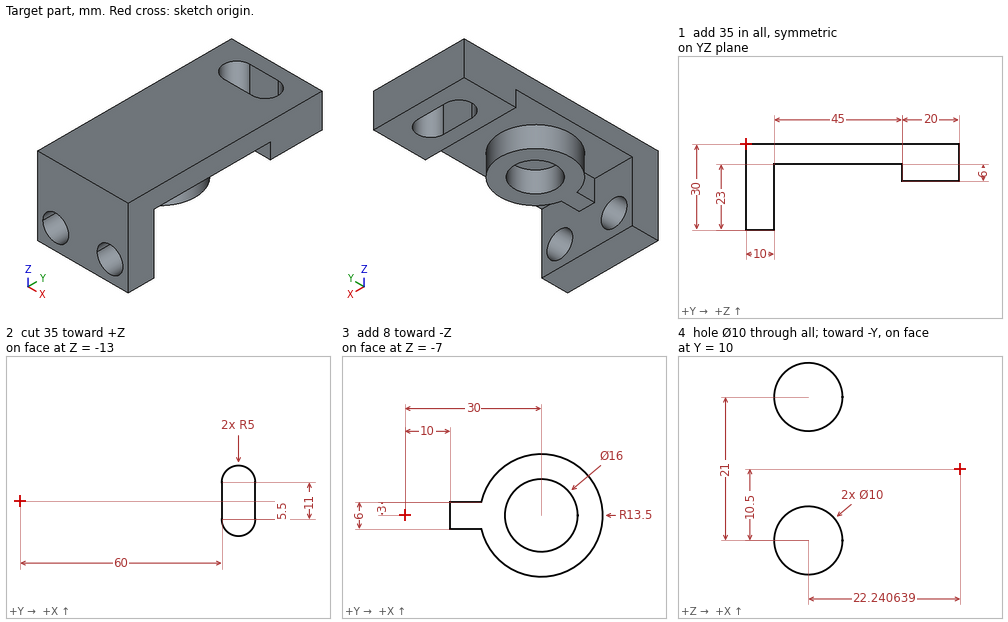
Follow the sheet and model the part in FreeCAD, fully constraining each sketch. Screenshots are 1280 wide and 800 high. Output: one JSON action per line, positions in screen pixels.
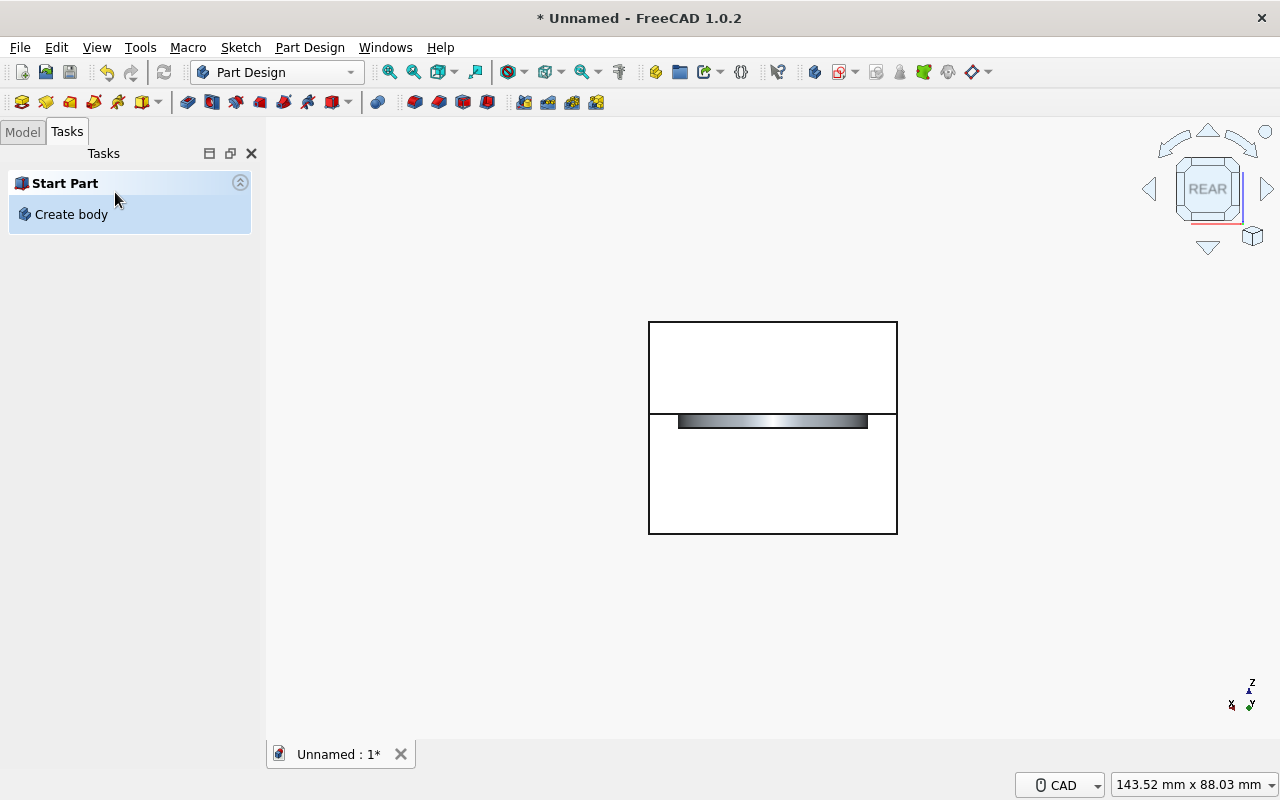
{"action": "key", "text": "v f"}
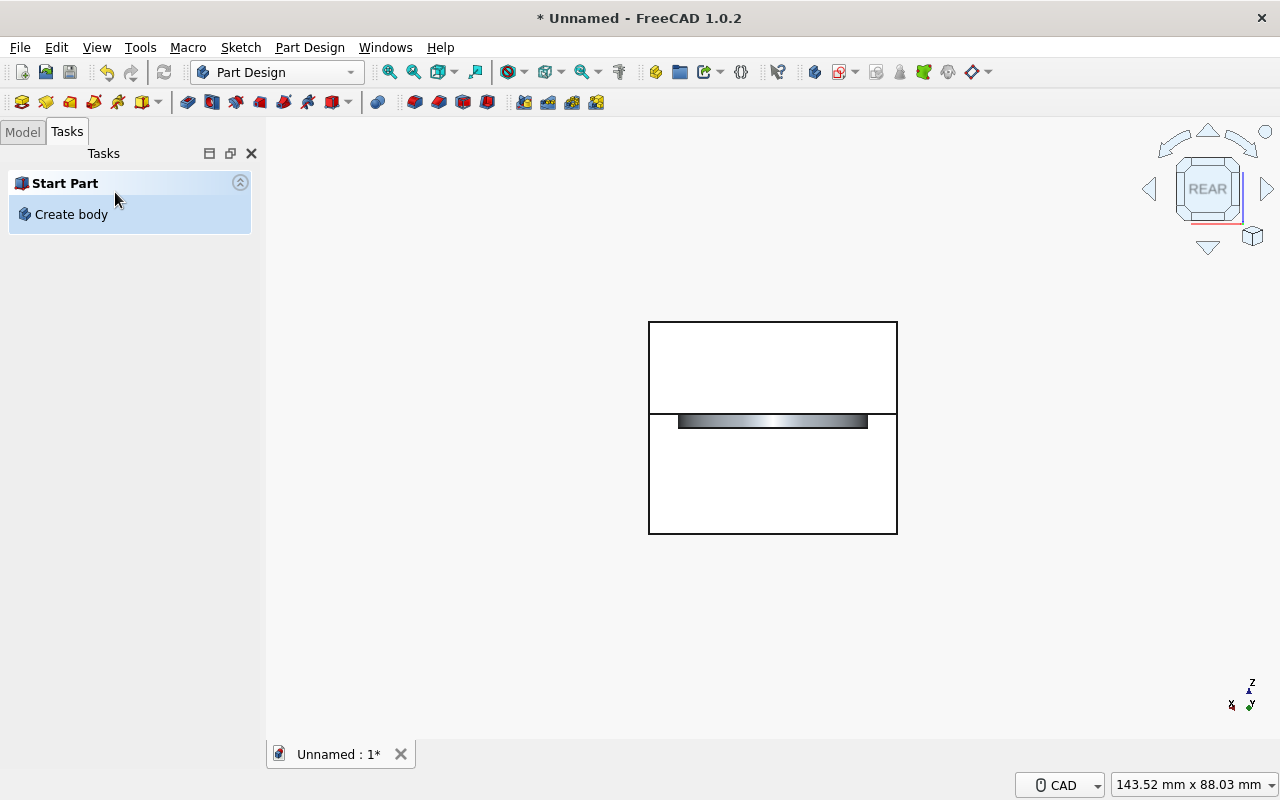
{"action": "left_click", "coordinate": [844, 475]}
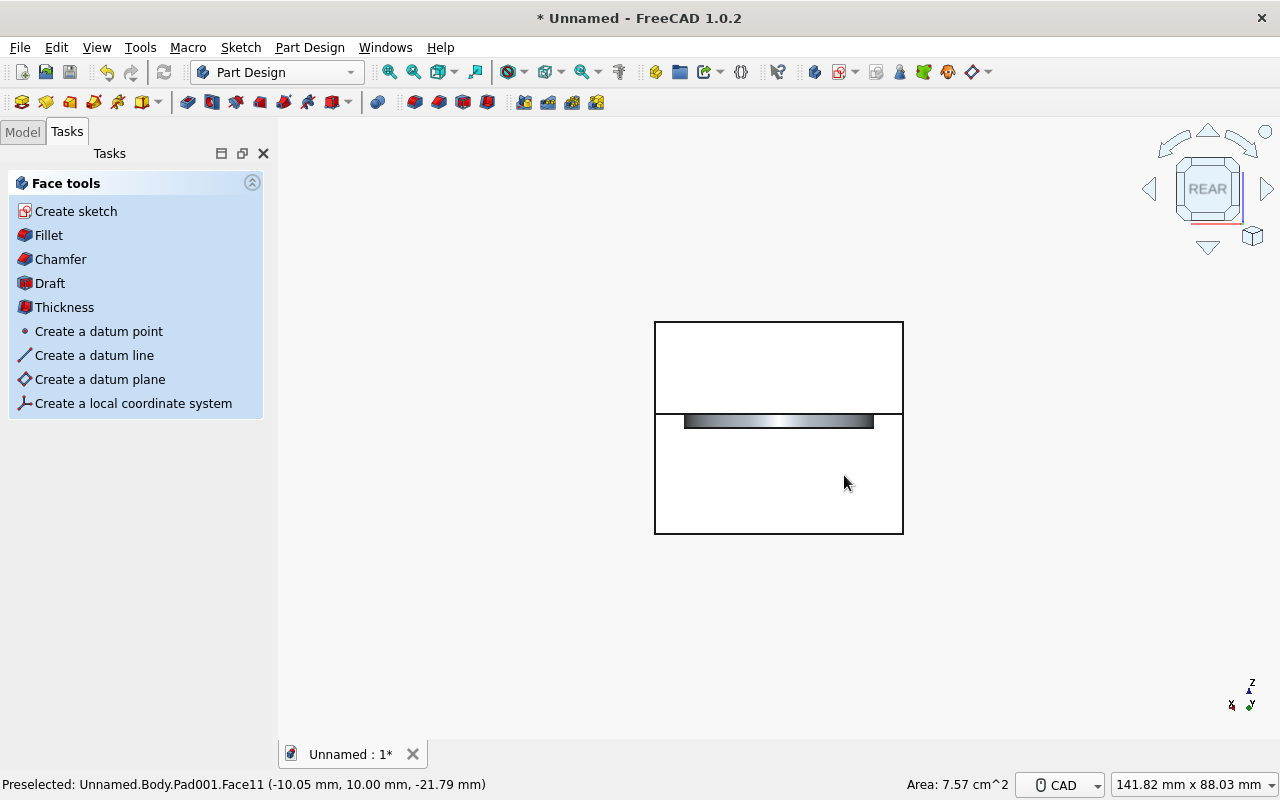
{"action": "left_click", "coordinate": [840, 72]}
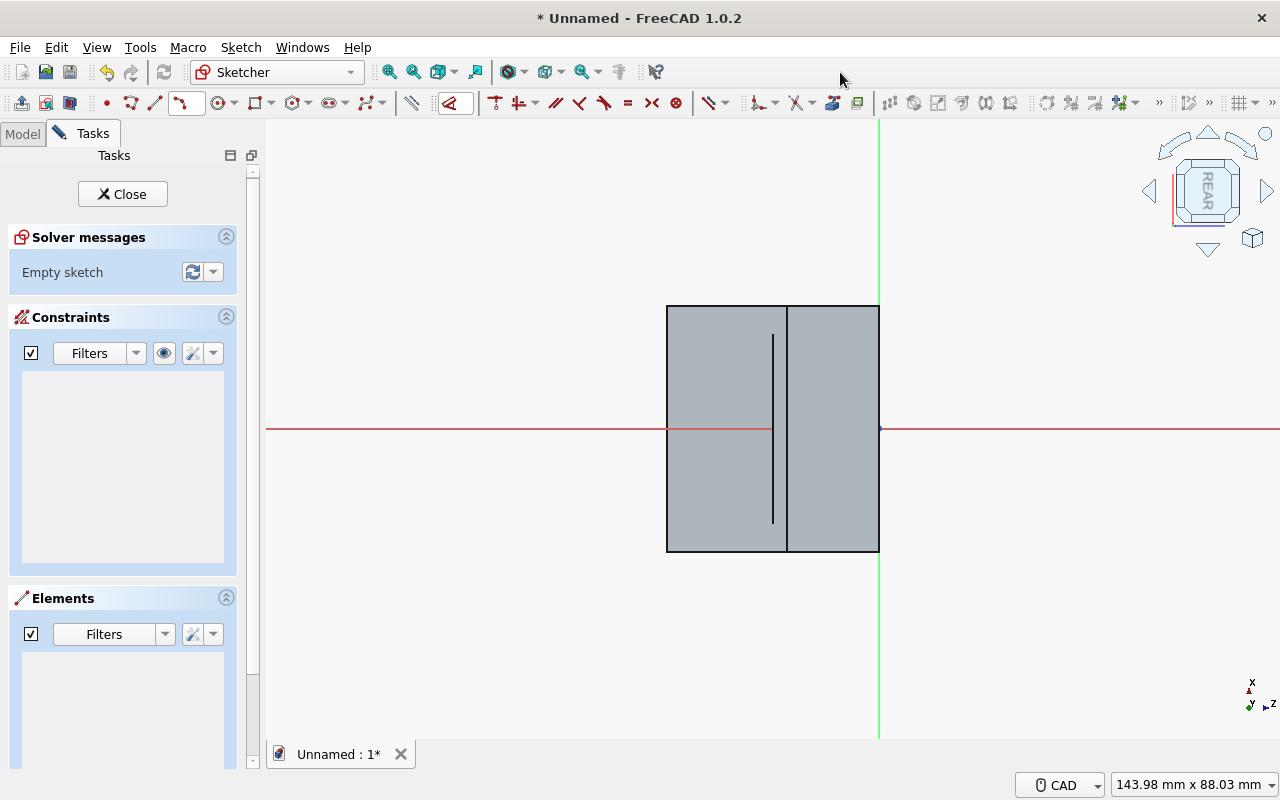
{"action": "left_click", "coordinate": [70, 104]}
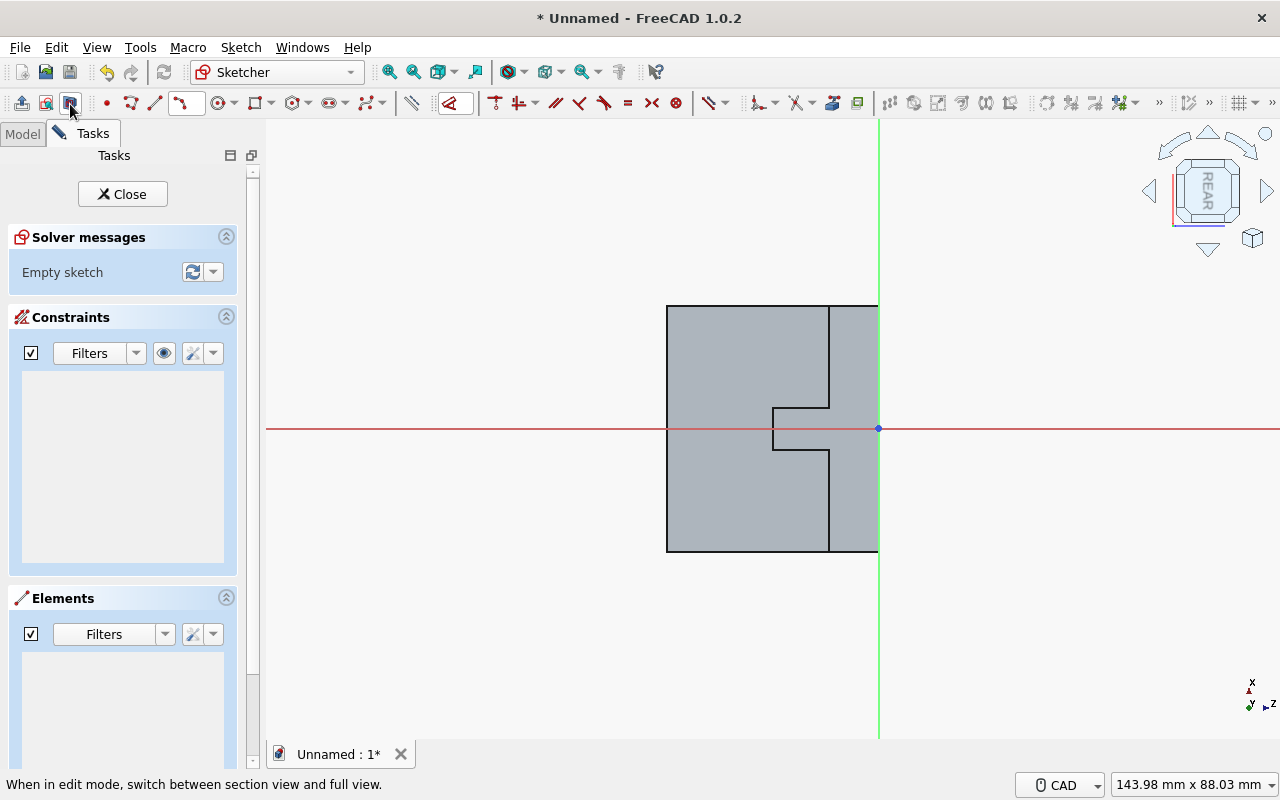
{"action": "scroll", "coordinate": [878, 429], "scroll_direction": "up", "scroll_amount": 3}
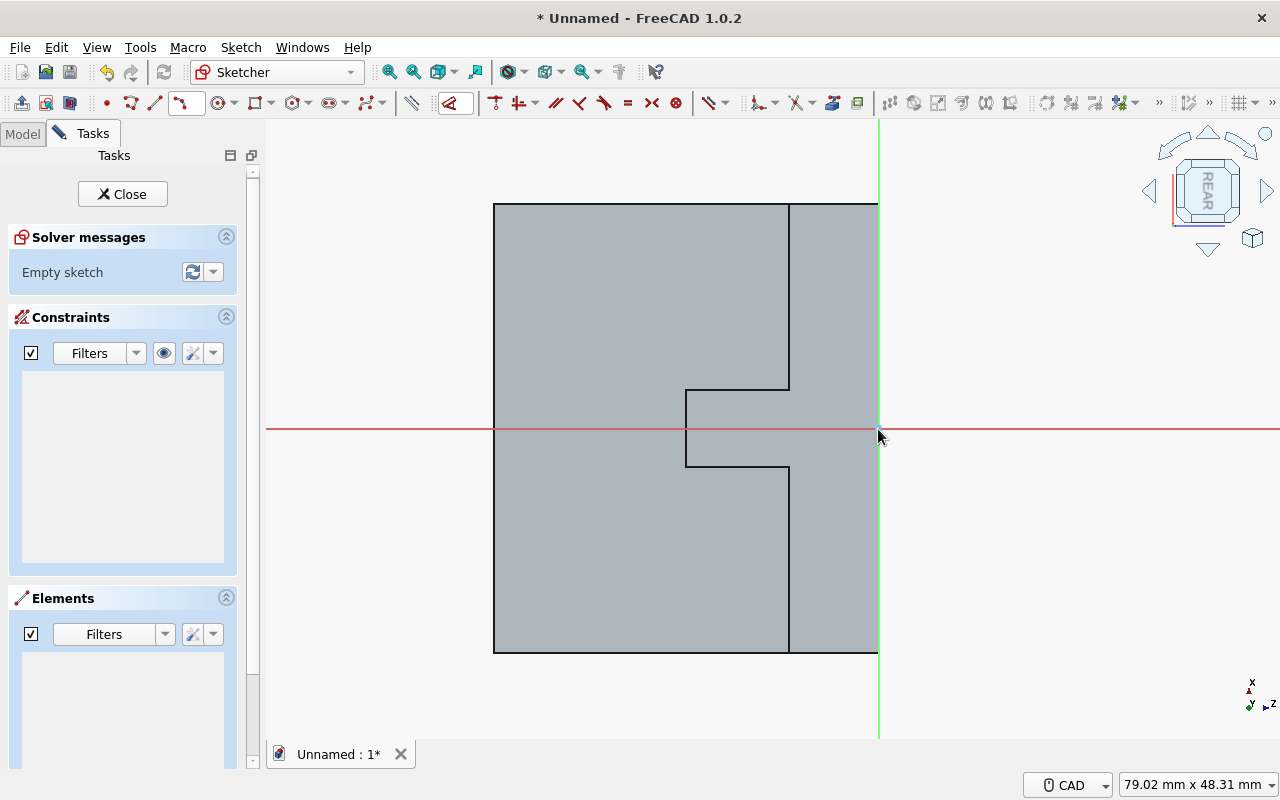
{"action": "left_click", "coordinate": [218, 104]}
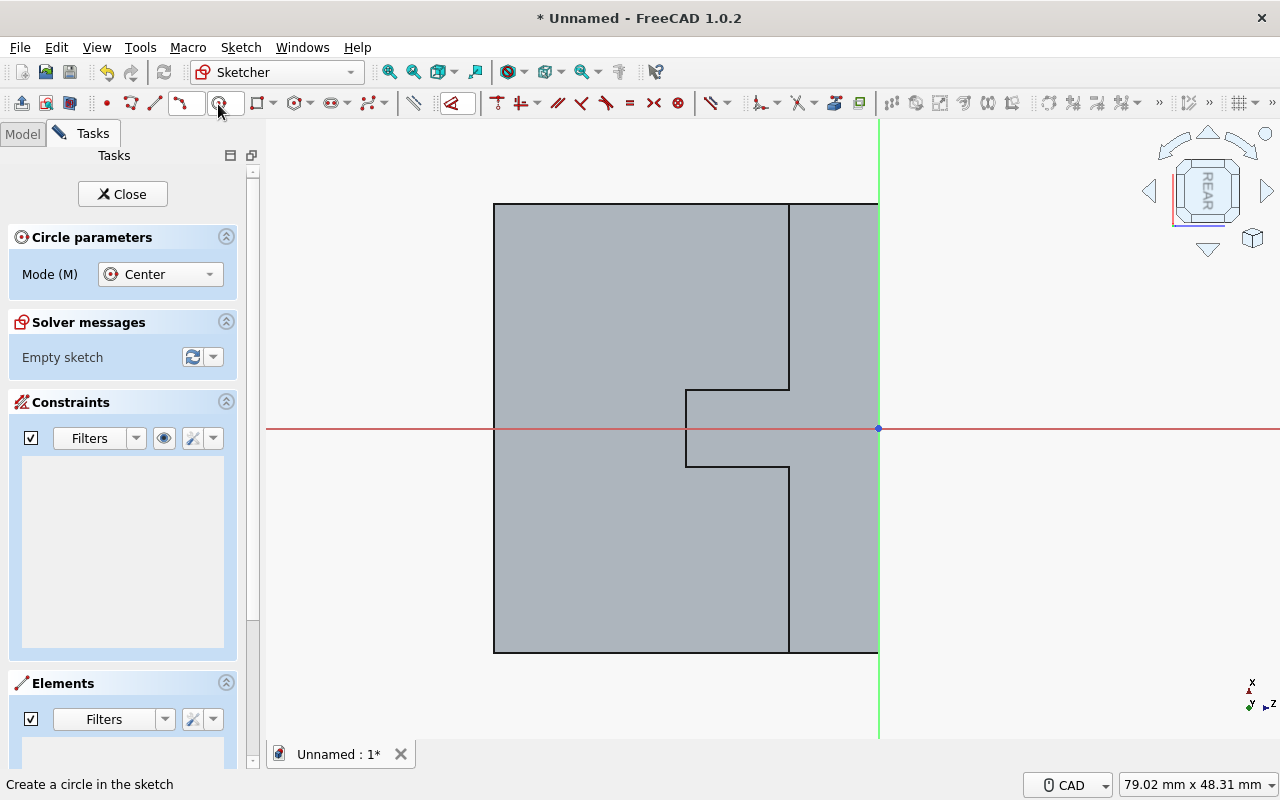
{"action": "left_click", "coordinate": [593, 563]}
{"action": "mouse_move", "coordinate": [639, 518]}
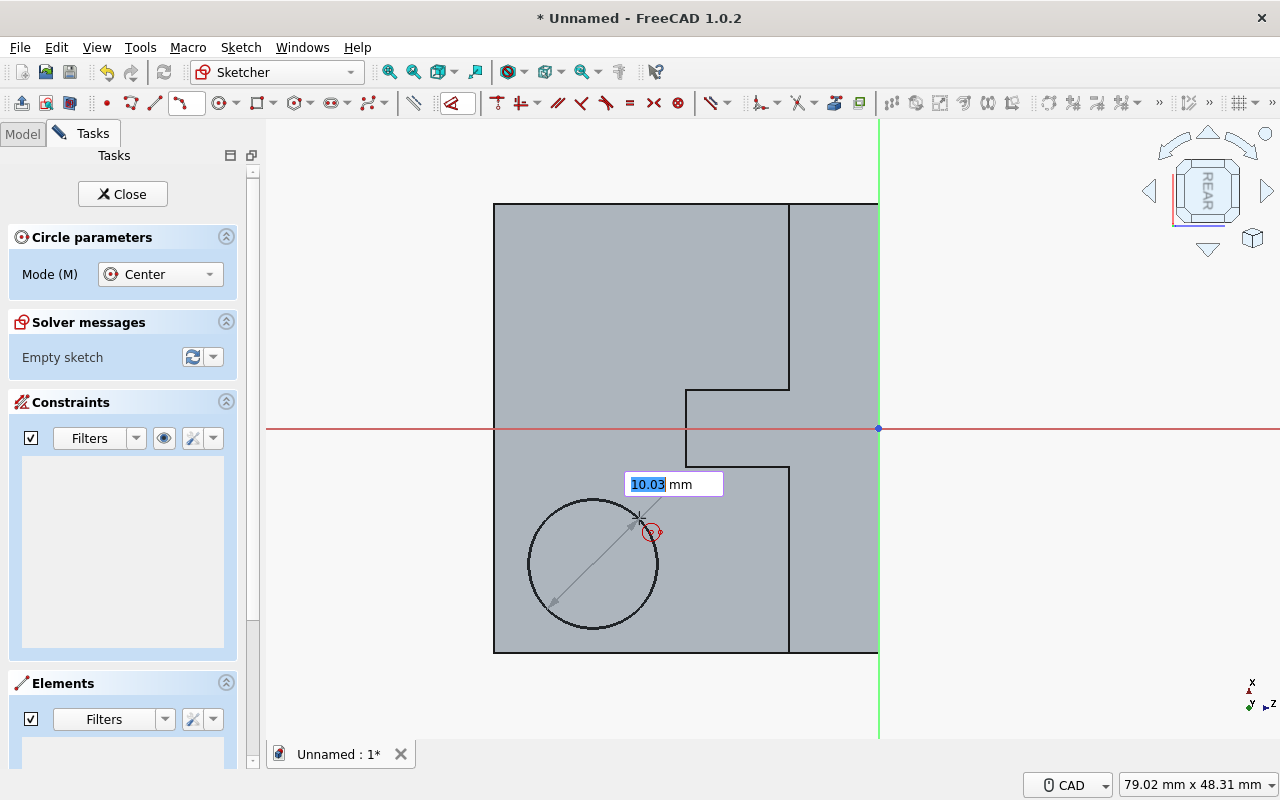
{"action": "type", "text": "10"}
{"action": "key", "text": "Return"}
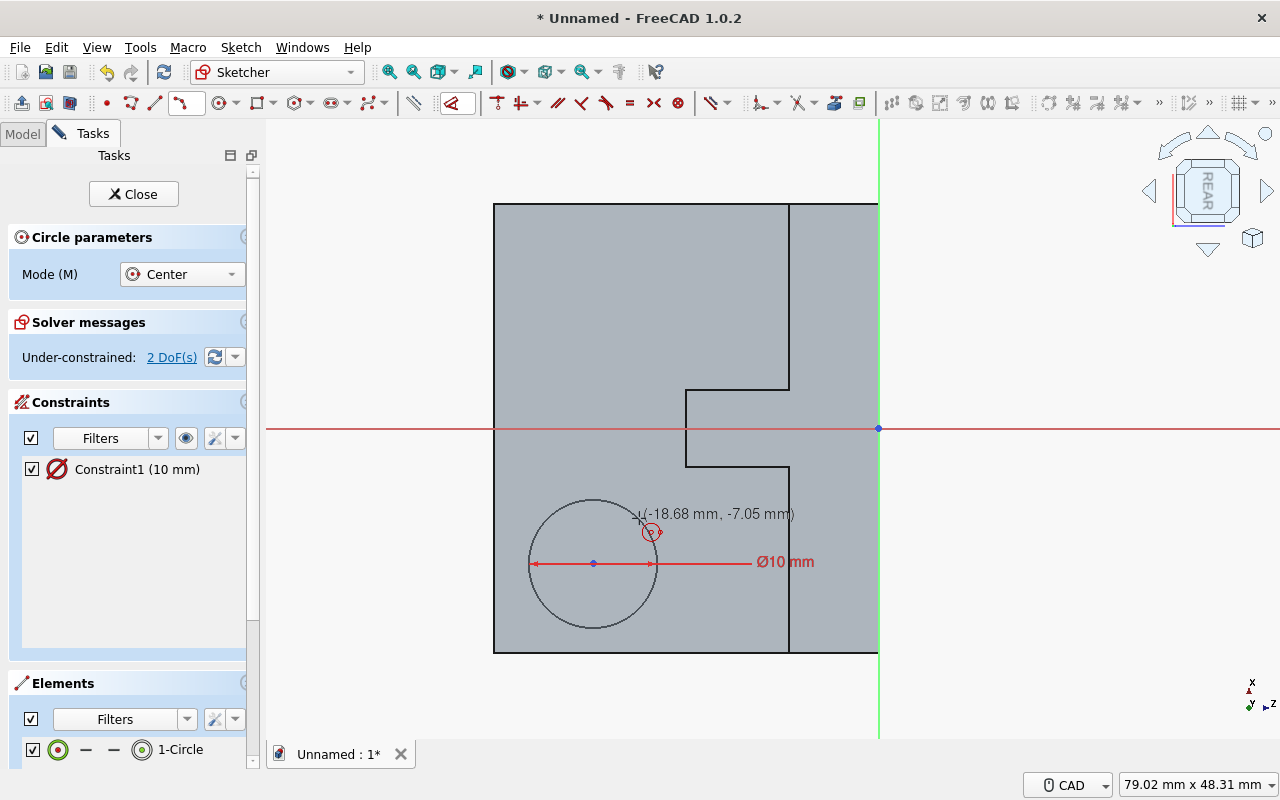
{"action": "left_click", "coordinate": [593, 294]}
{"action": "mouse_move", "coordinate": [639, 248]}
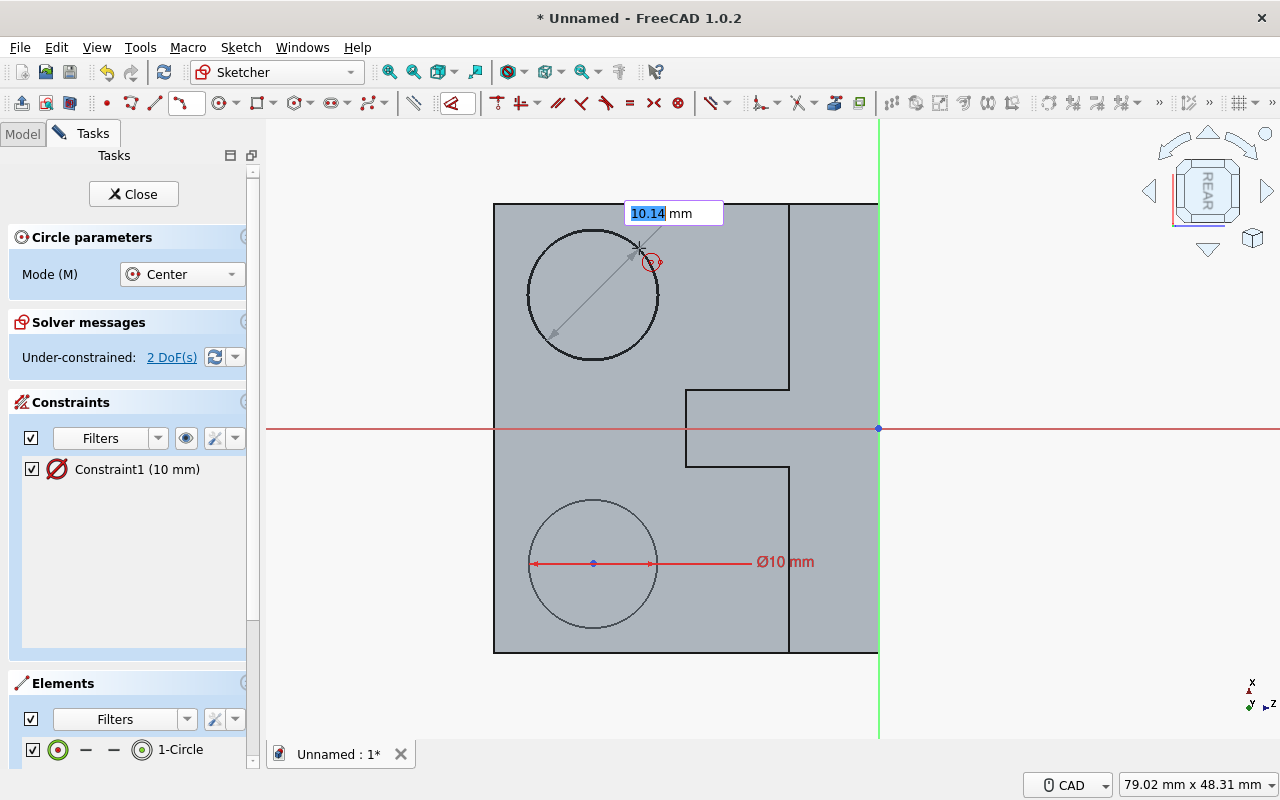
{"action": "type", "text": "10"}
{"action": "key", "text": "Return"}
{"action": "key", "text": "Escape"}